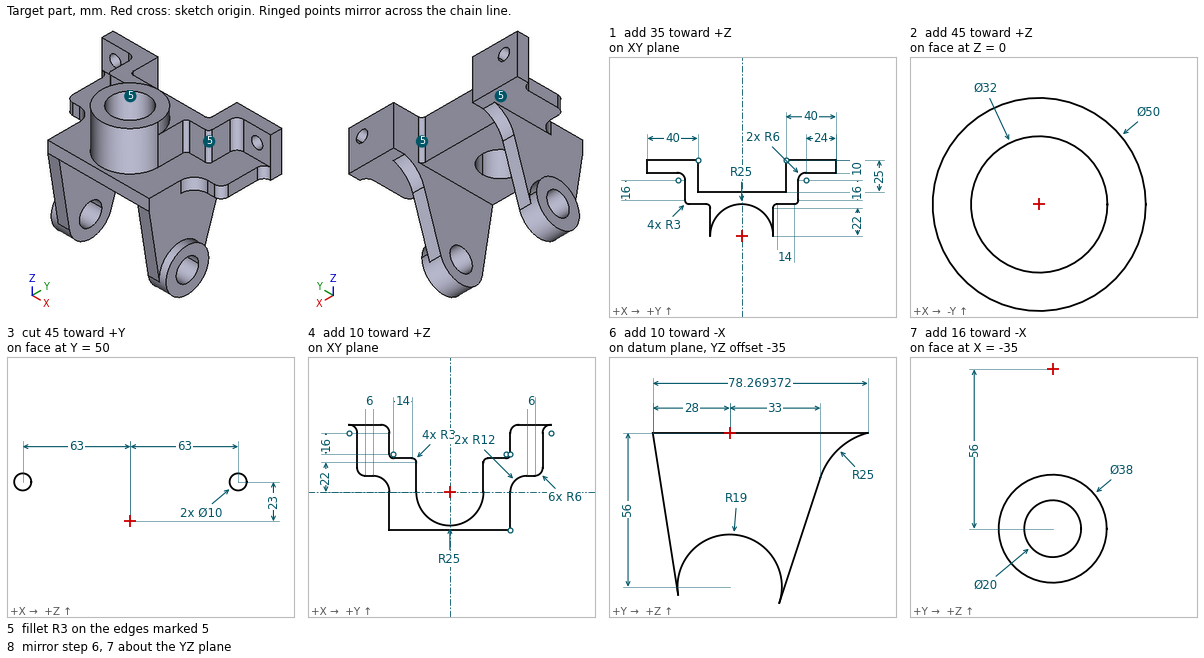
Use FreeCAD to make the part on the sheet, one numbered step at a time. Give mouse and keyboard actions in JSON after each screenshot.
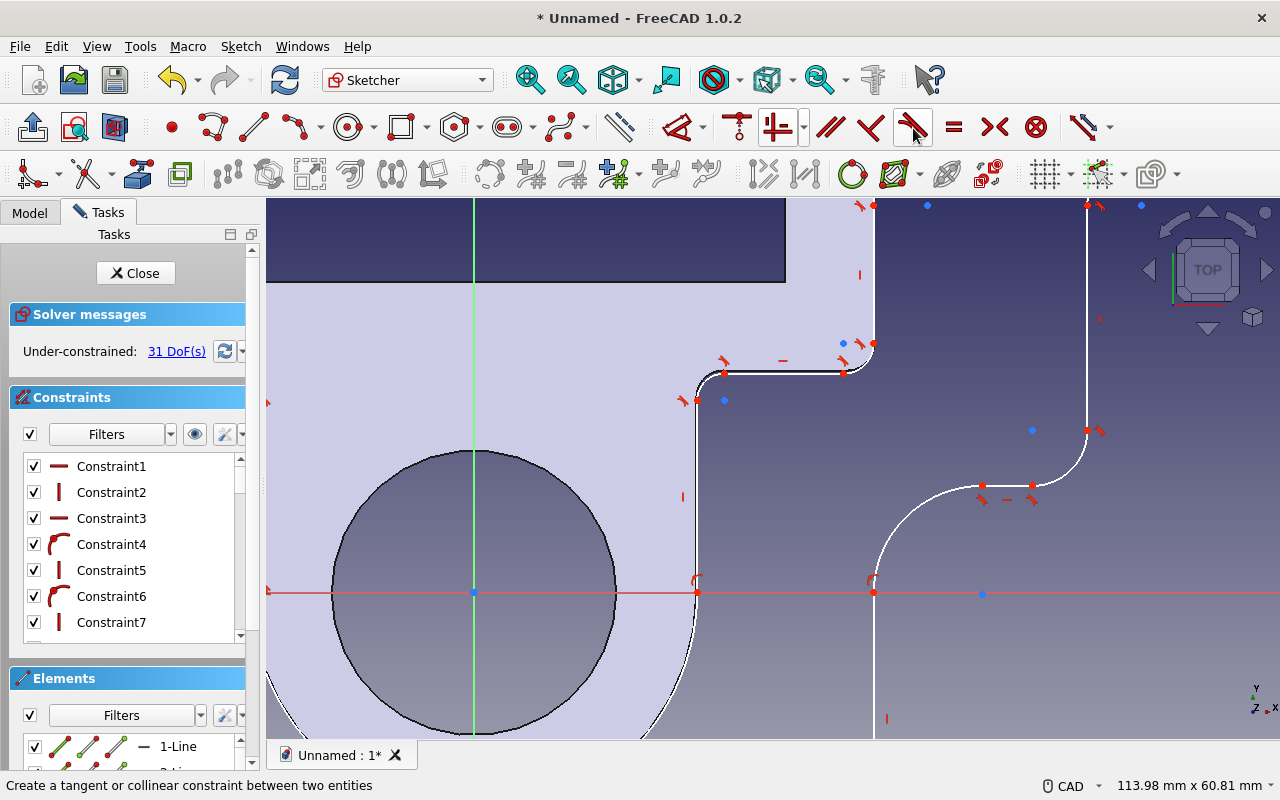
{"action": "left_click", "coordinate": [874, 668]}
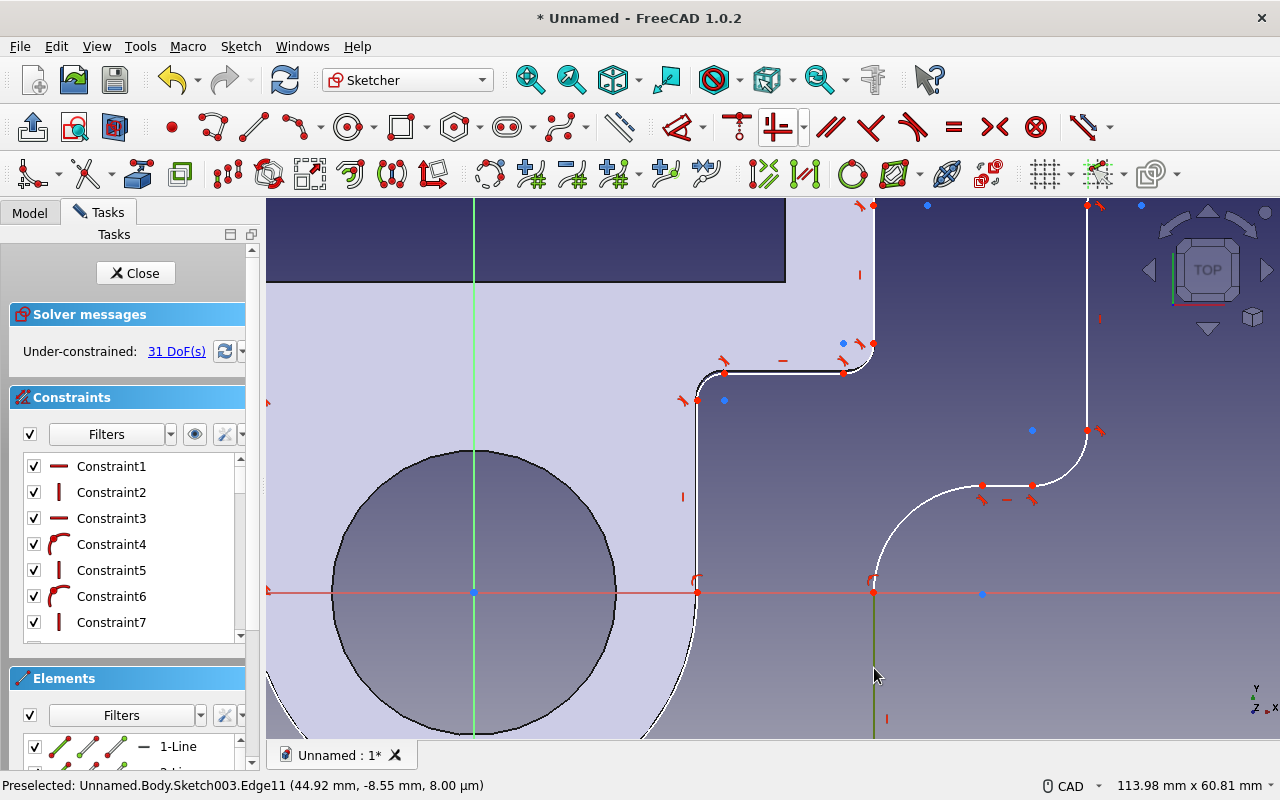
{"action": "left_click", "coordinate": [933, 498]}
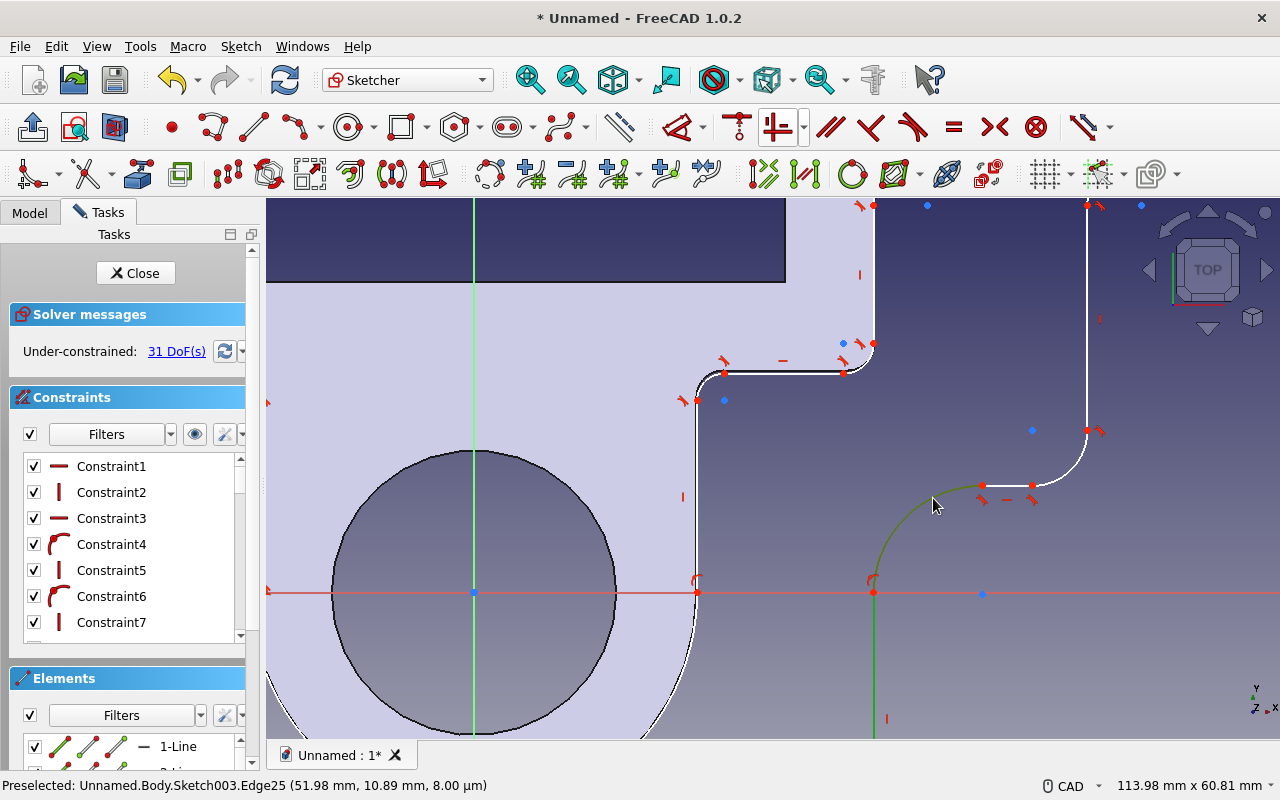
{"action": "left_click", "coordinate": [913, 128]}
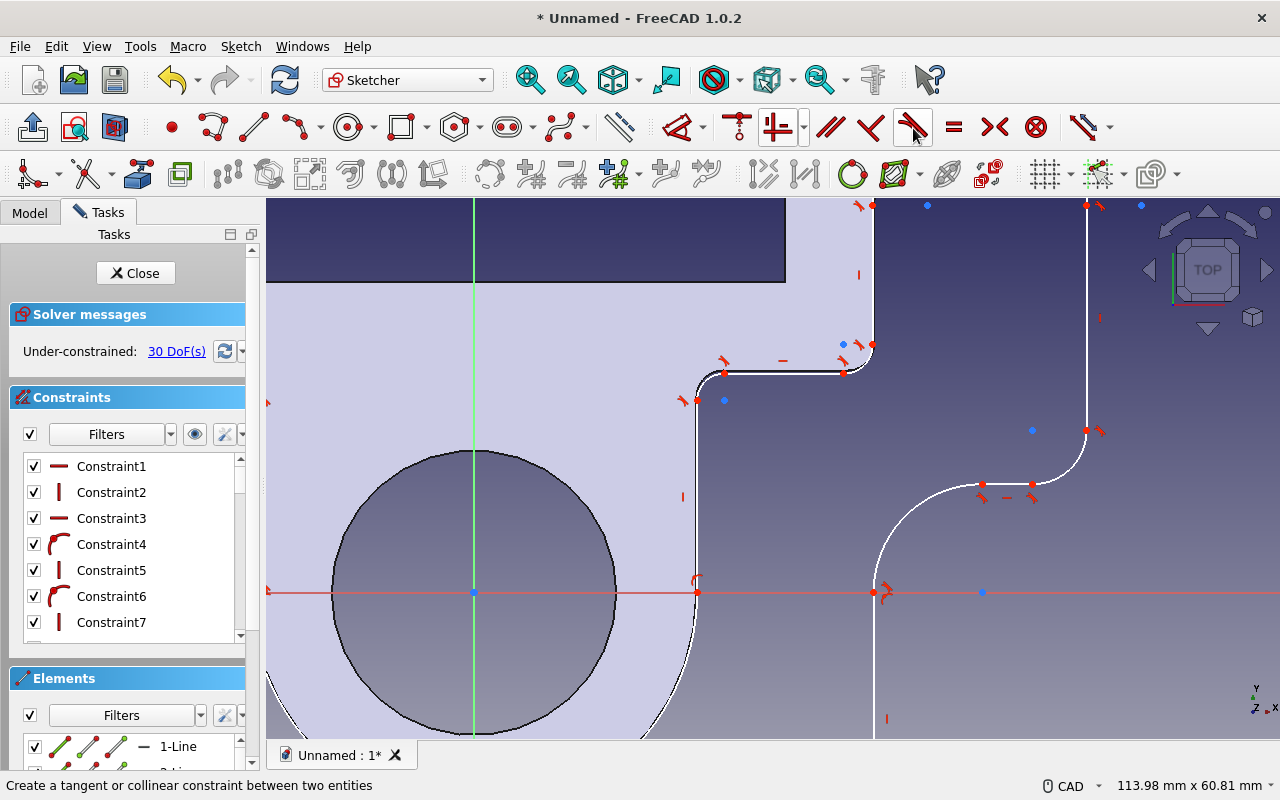
{"action": "scroll", "coordinate": [893, 447], "scroll_direction": "down", "scroll_amount": 4}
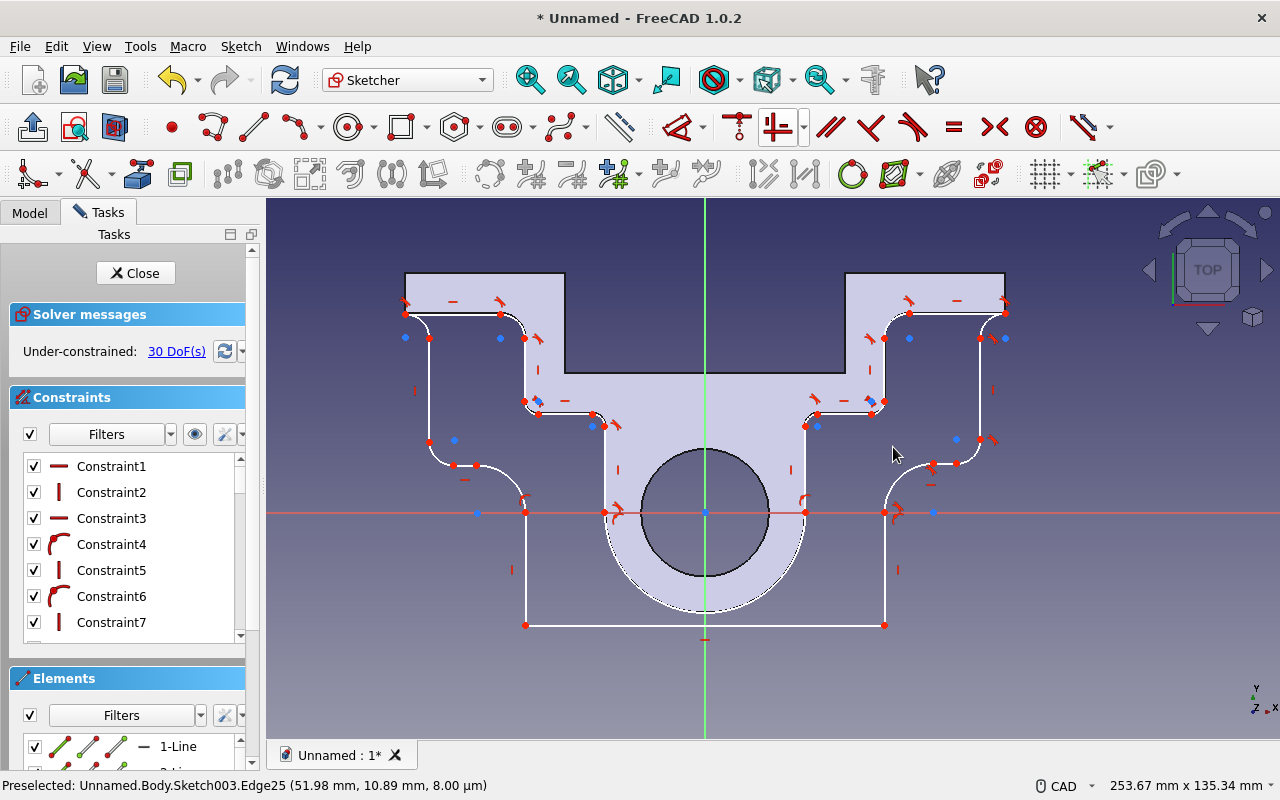
{"action": "left_click", "coordinate": [526, 592]}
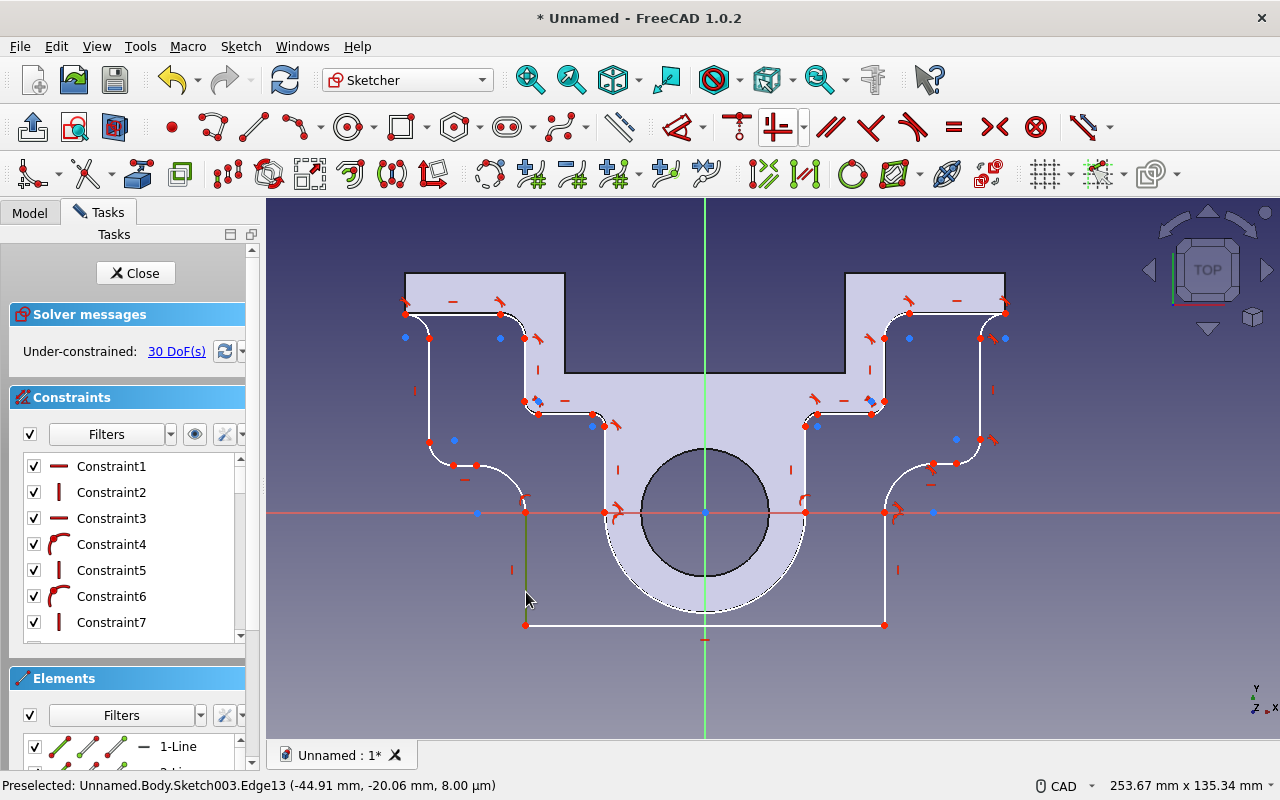
{"action": "left_click", "coordinate": [520, 491]}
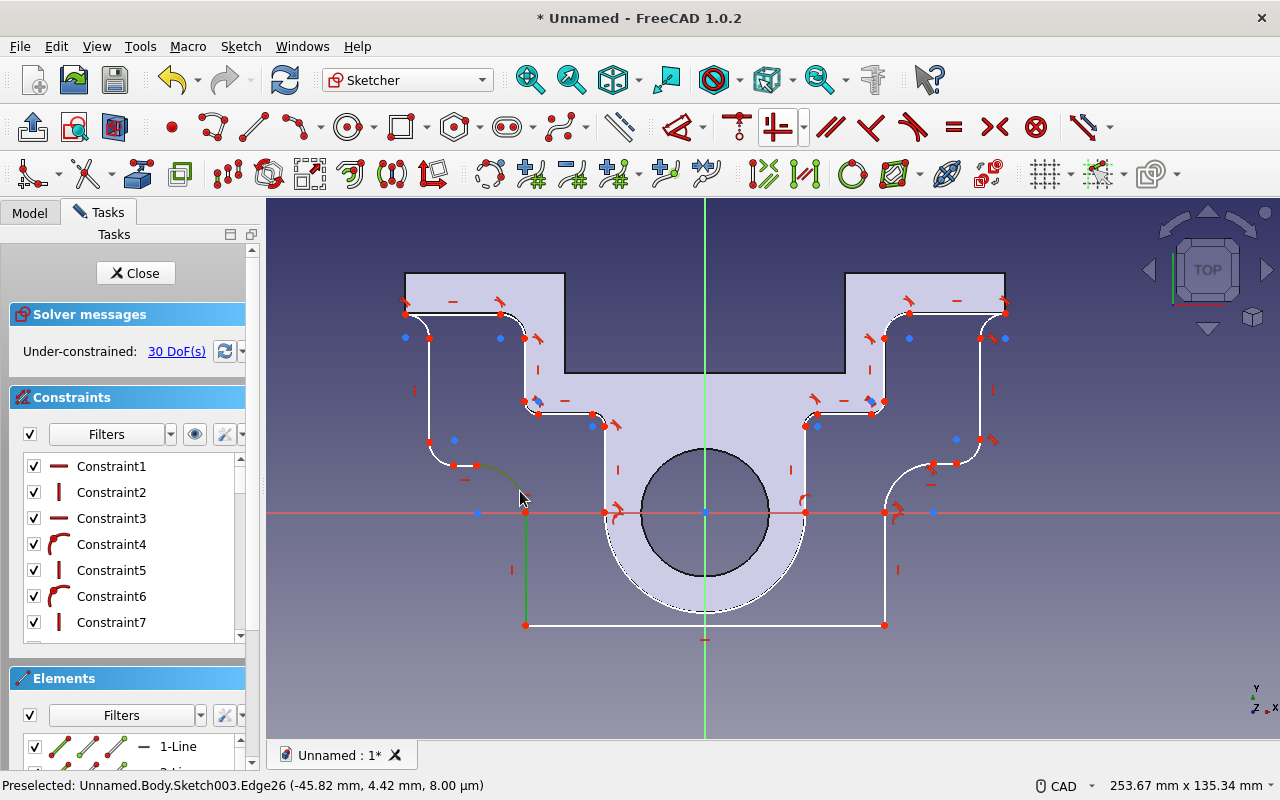
{"action": "left_click", "coordinate": [913, 128]}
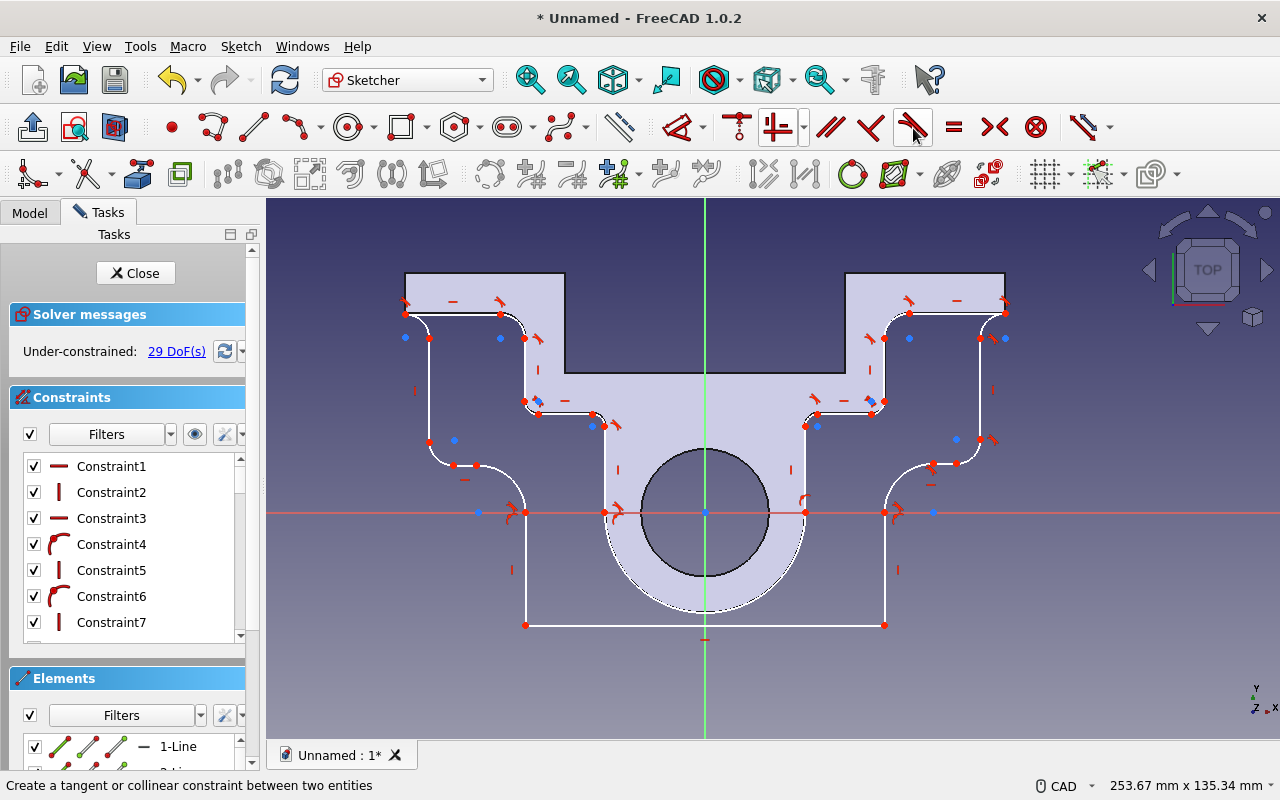
{"action": "scroll", "coordinate": [467, 466], "scroll_direction": "up", "scroll_amount": 2}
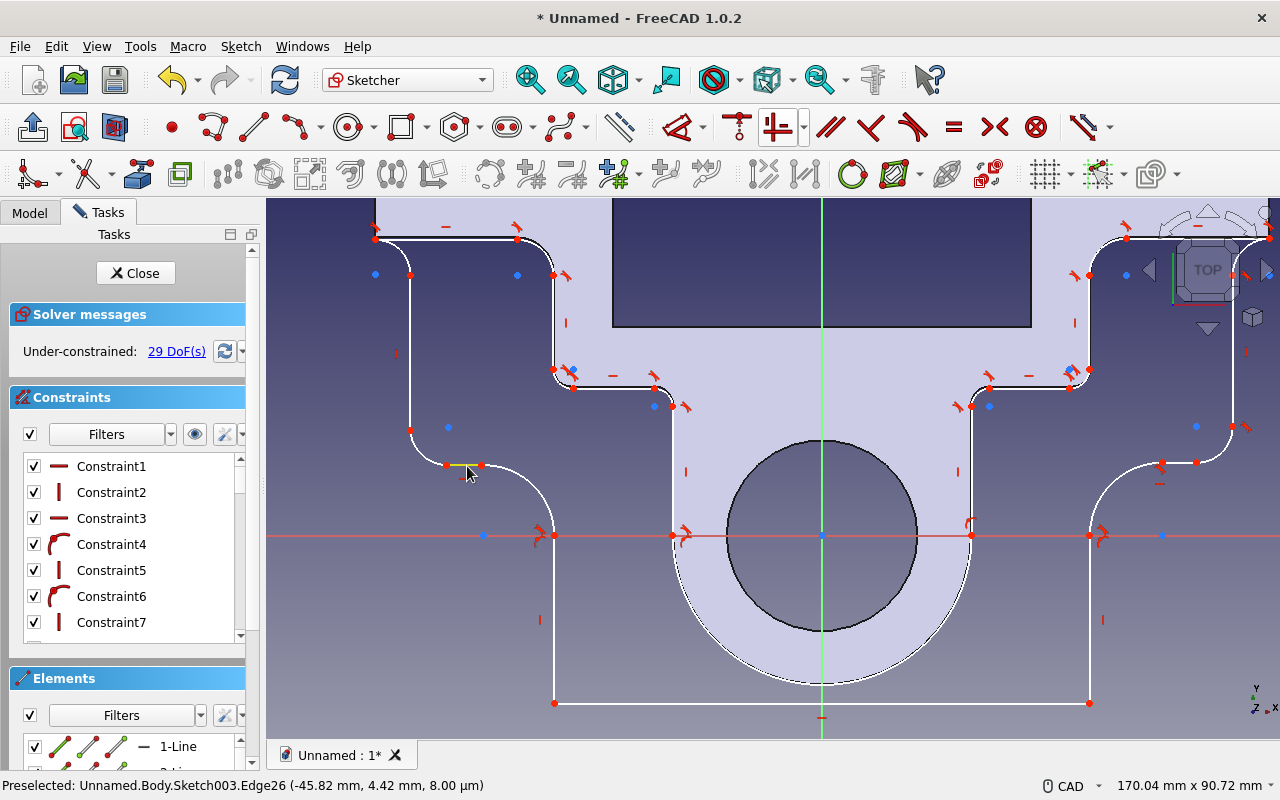
{"action": "left_click", "coordinate": [467, 465]}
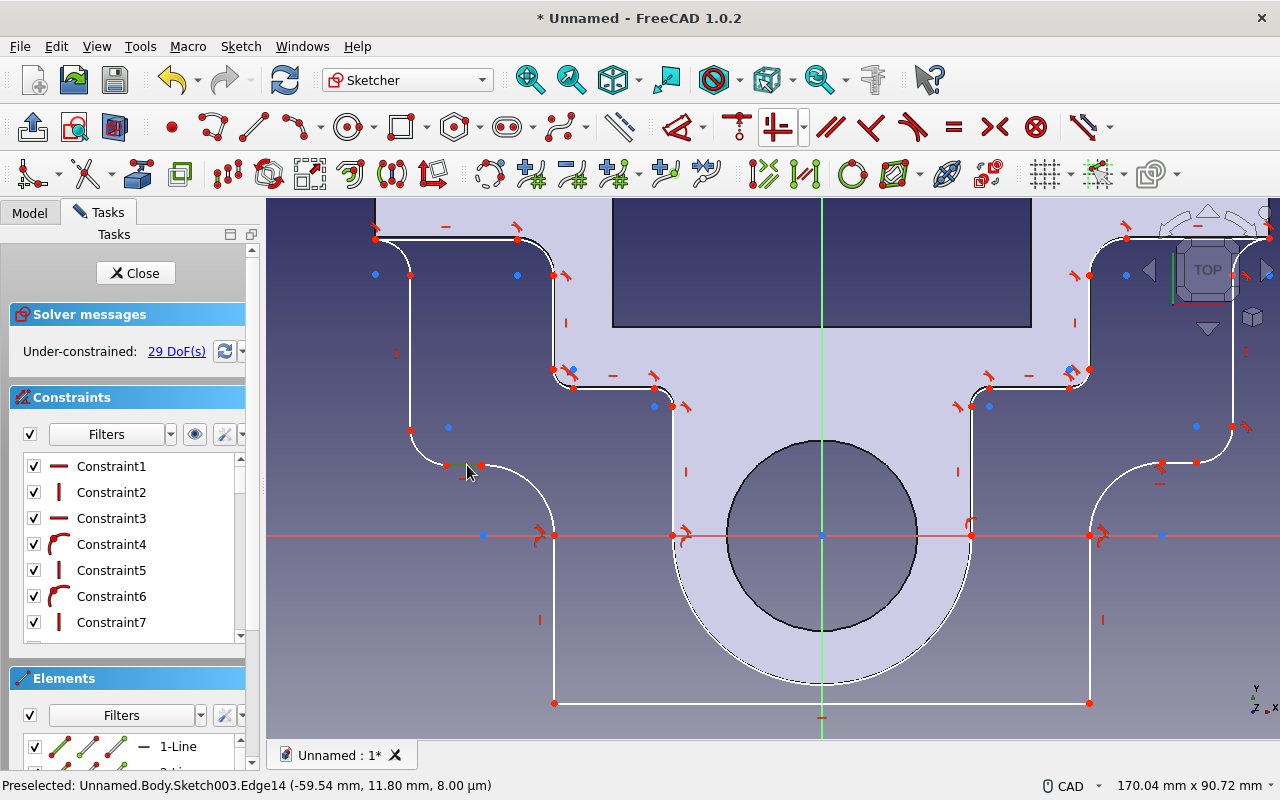
{"action": "left_click", "coordinate": [546, 503]}